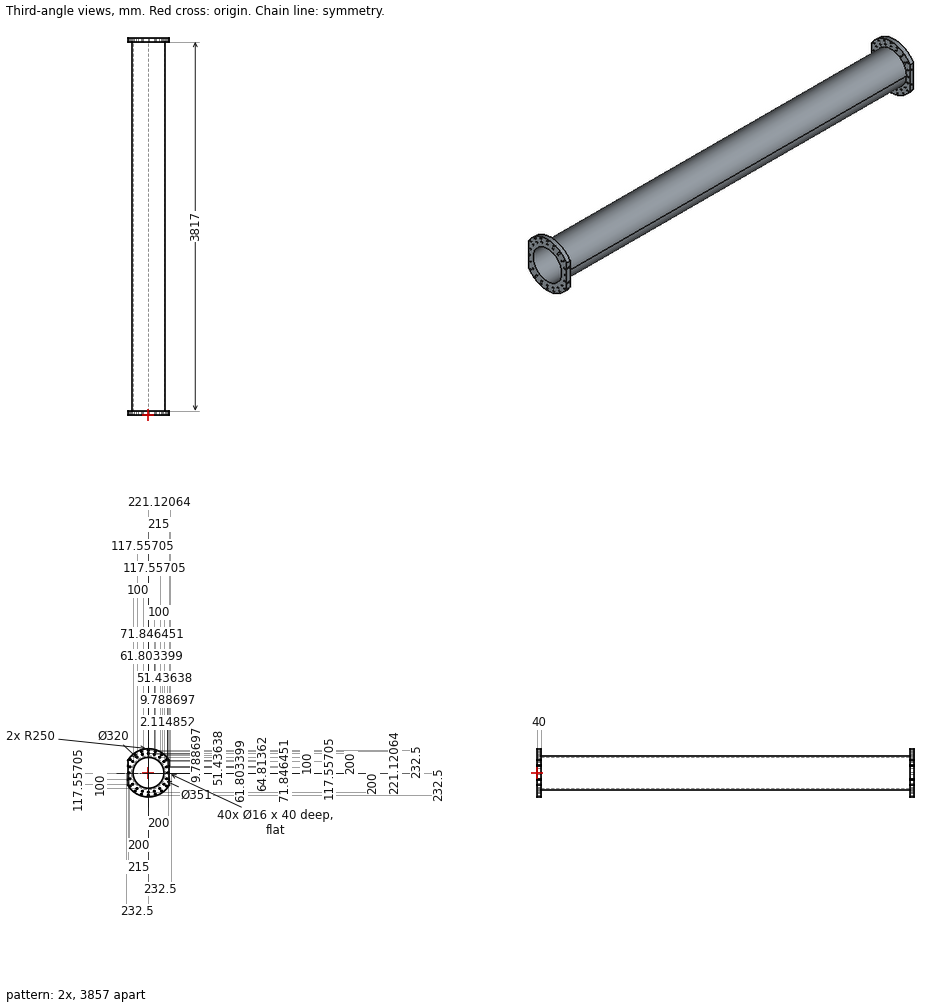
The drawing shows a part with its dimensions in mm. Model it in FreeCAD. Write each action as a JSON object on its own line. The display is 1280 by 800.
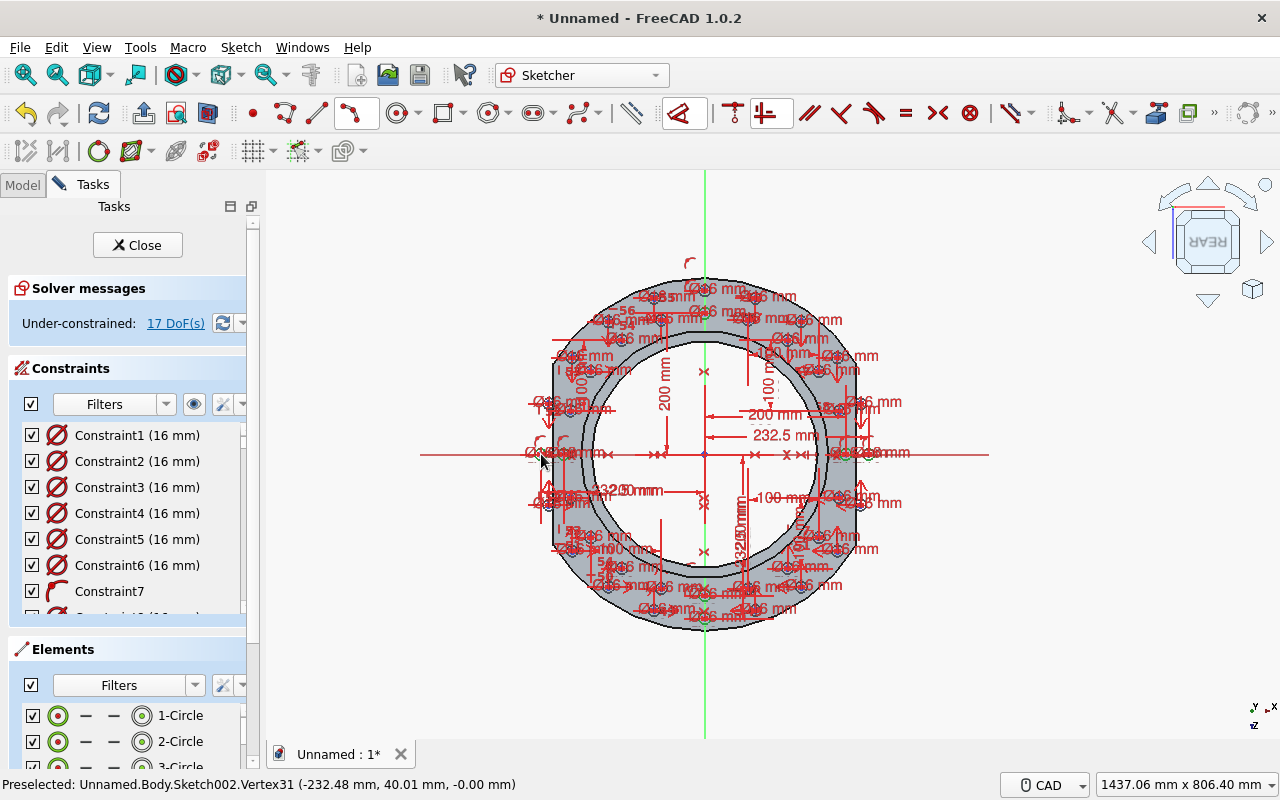
{"action": "left_click", "coordinate": [705, 291]}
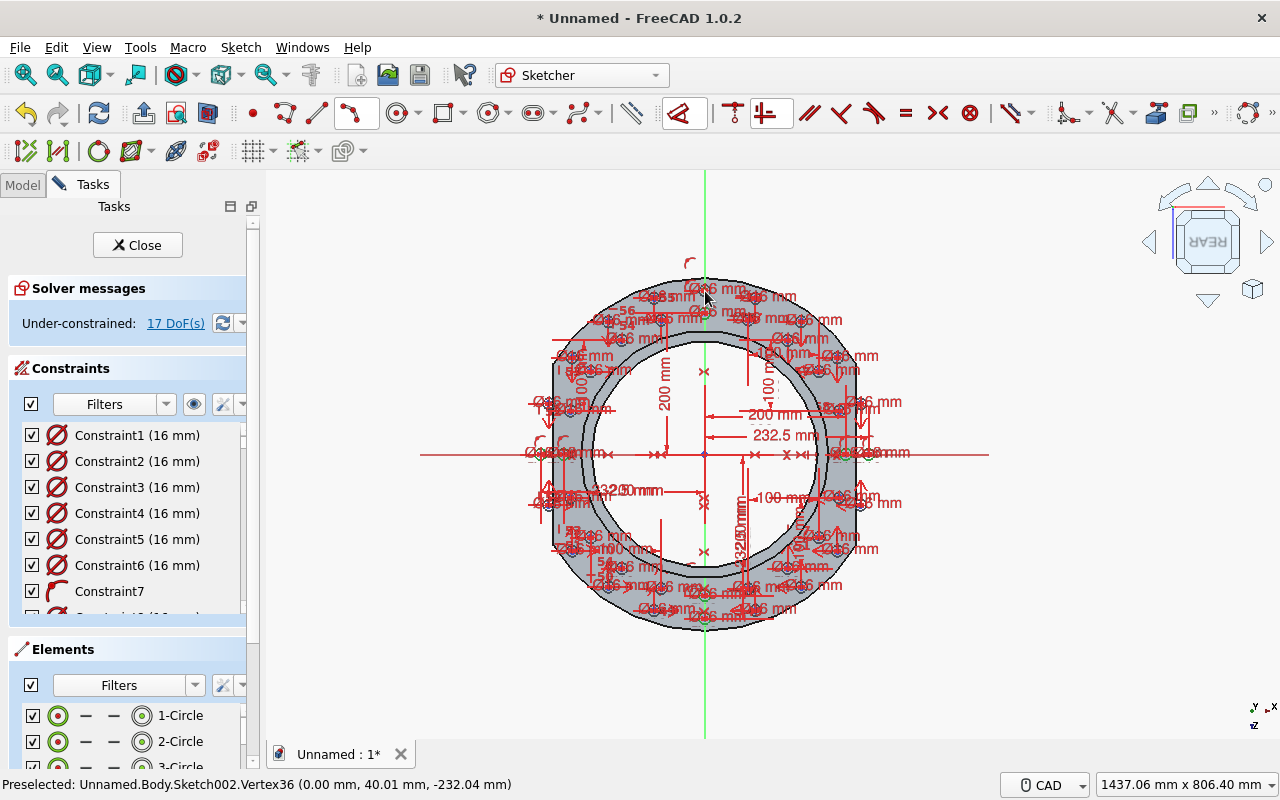
{"action": "key", "text": "i"}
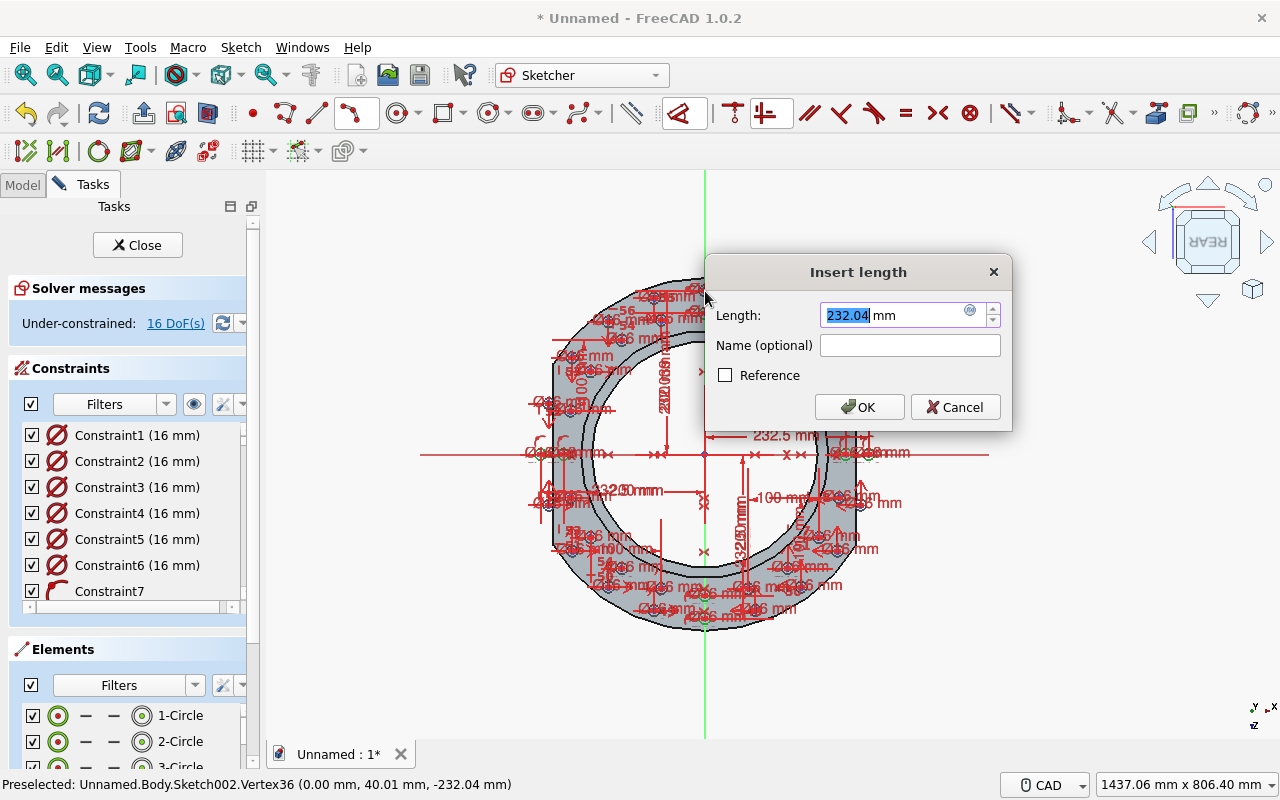
{"action": "type", "text": "232.5"}
{"action": "key", "text": "Return"}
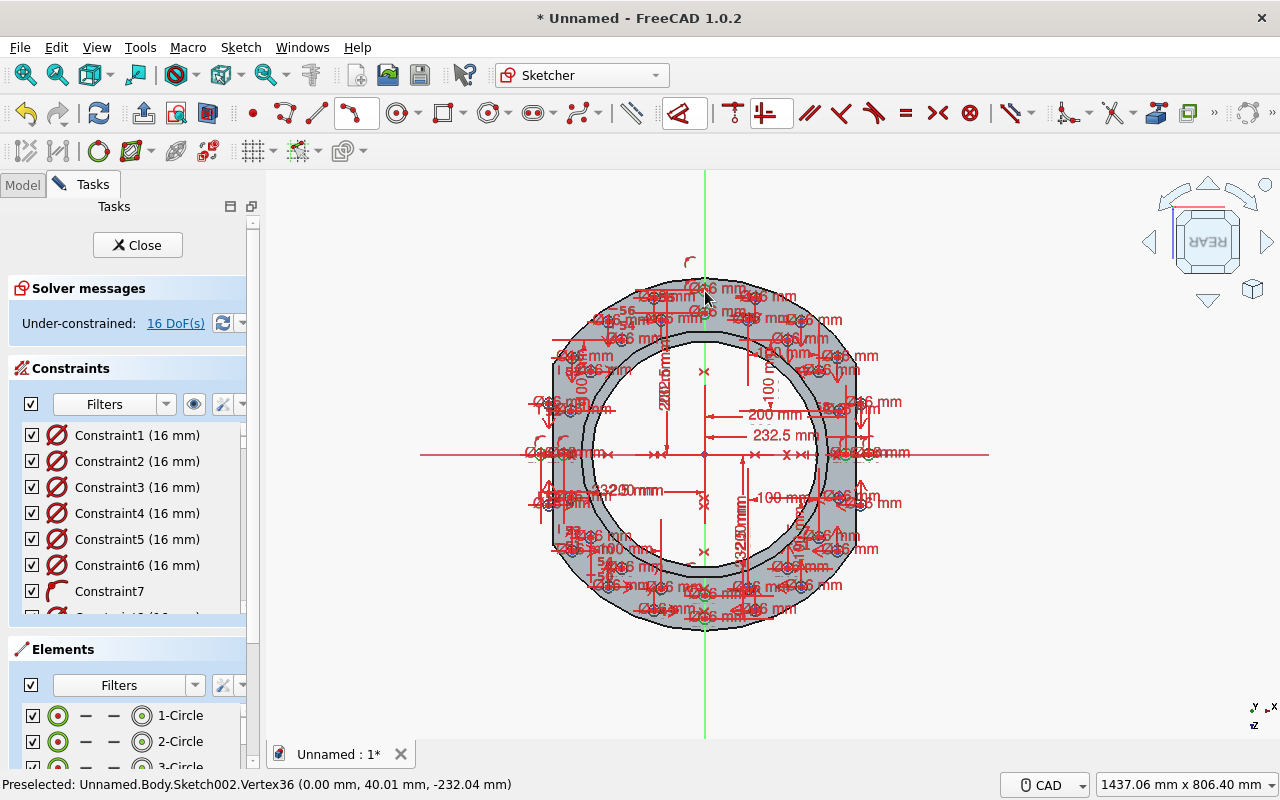
{"action": "left_click", "coordinate": [839, 498]}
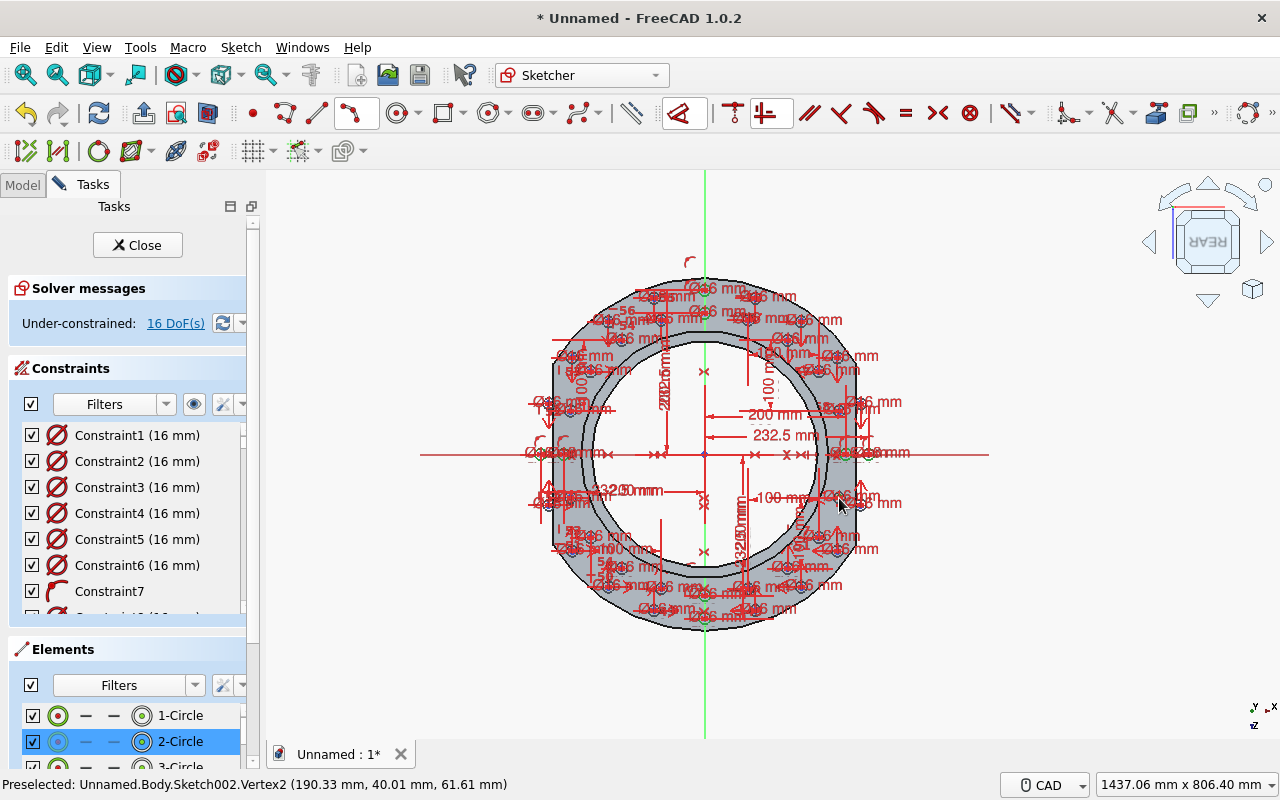
{"action": "key", "text": "i"}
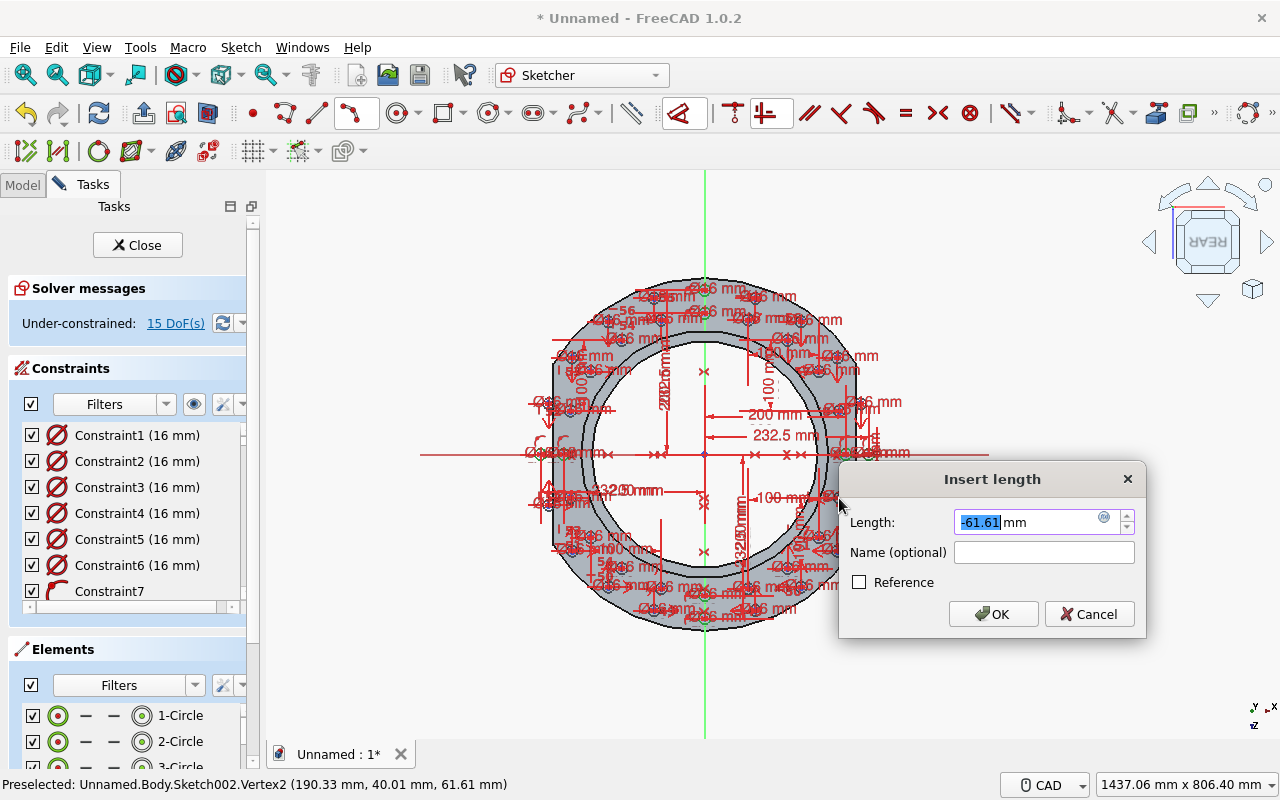
{"action": "type", "text": "-61.803399"}
{"action": "key", "text": "Return"}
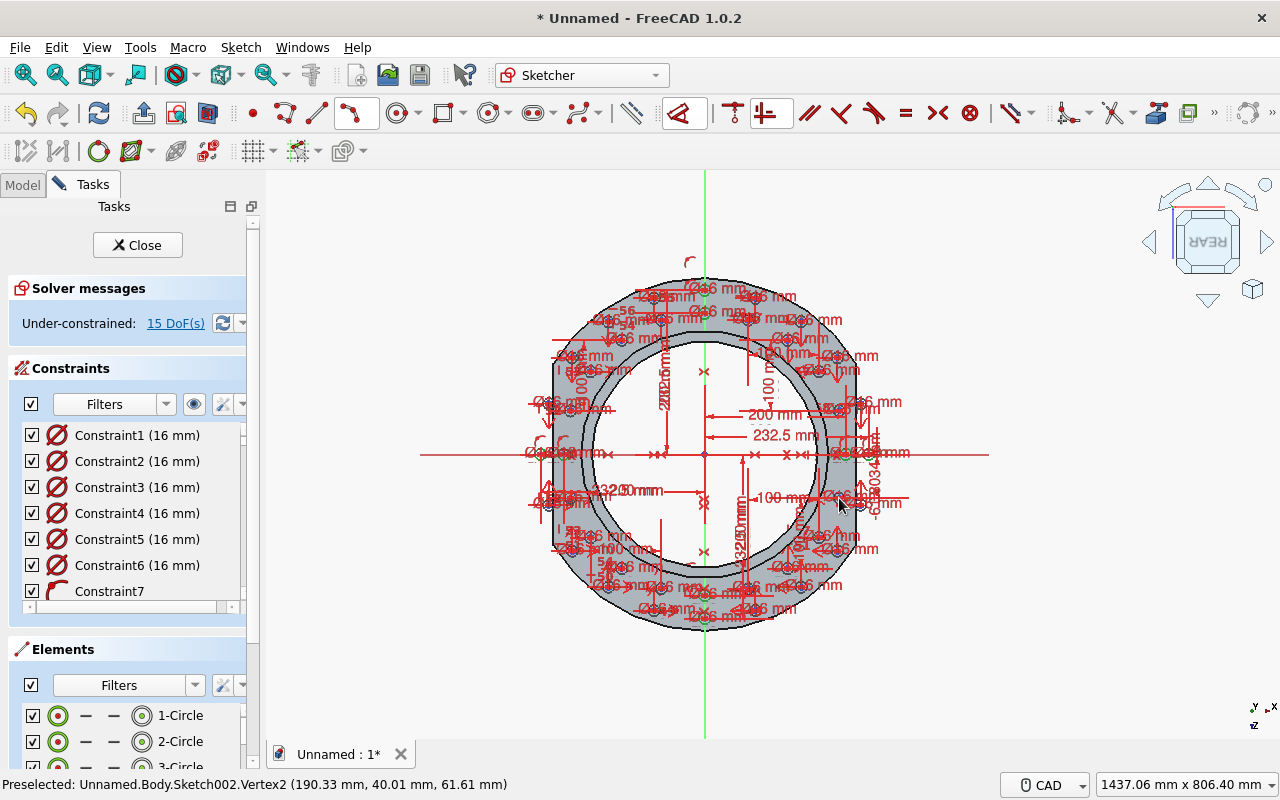
{"action": "left_click", "coordinate": [819, 538]}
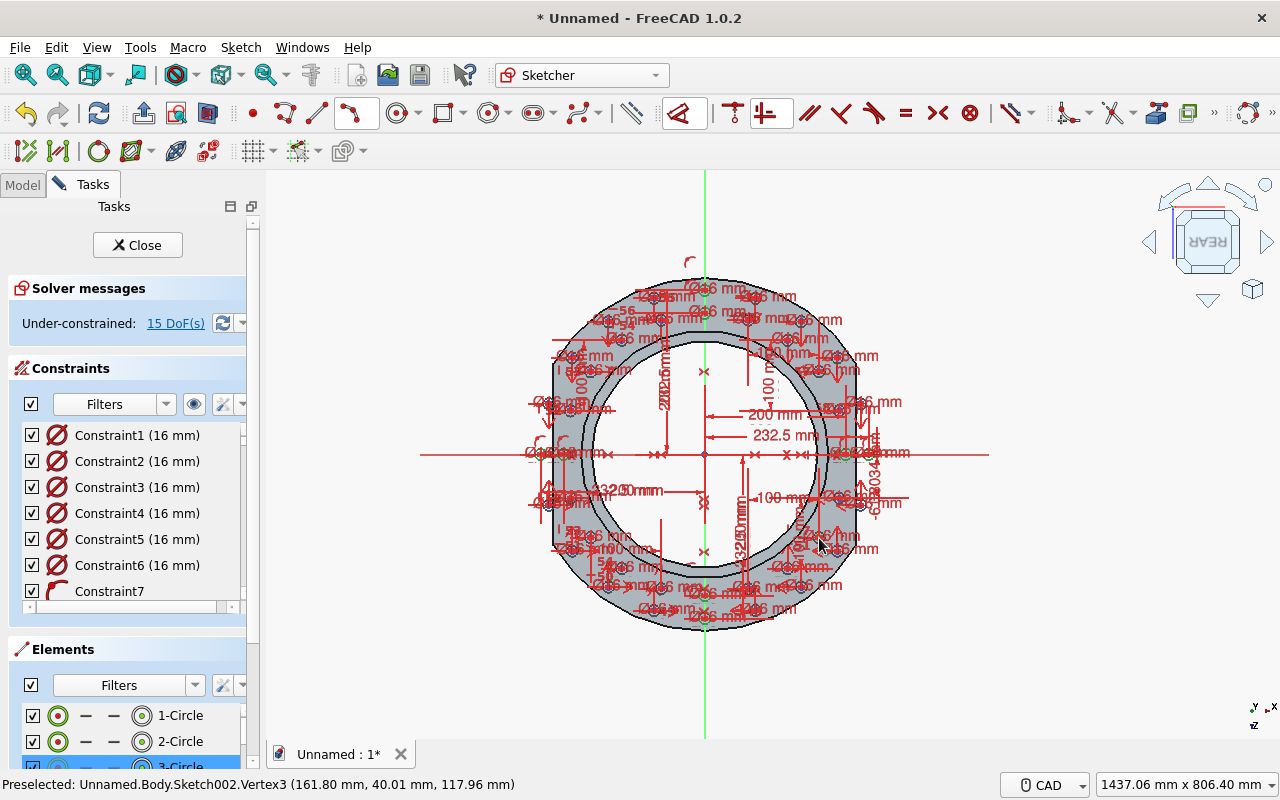
{"action": "key", "text": "i"}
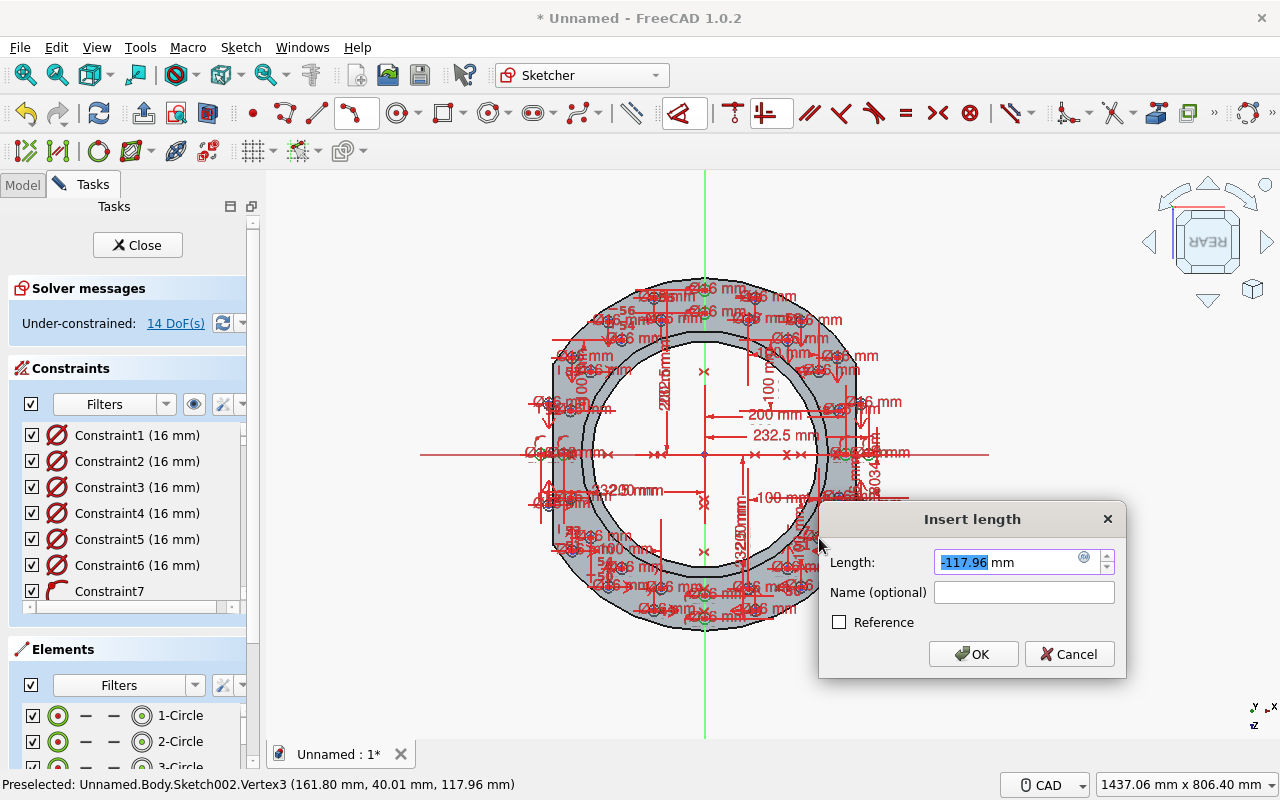
{"action": "type", "text": "-117.55705"}
{"action": "key", "text": "Return"}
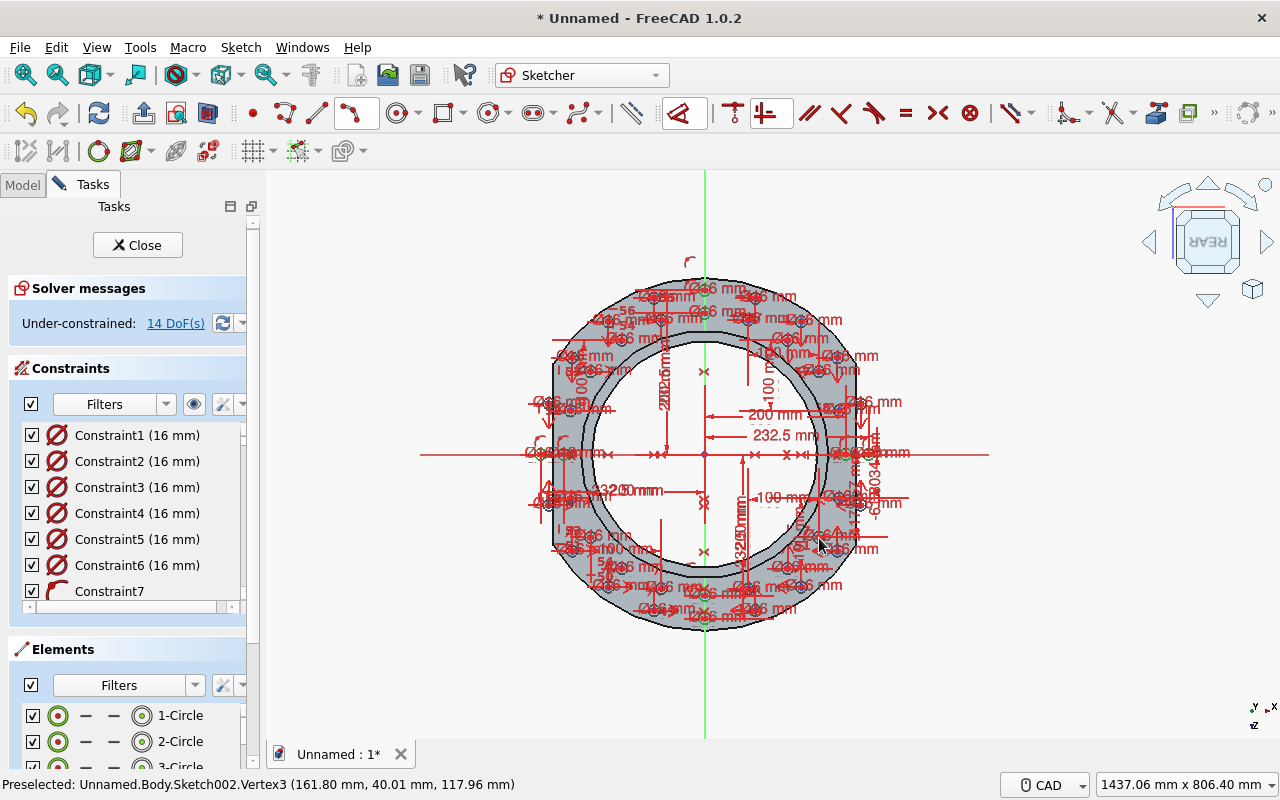
{"action": "left_click", "coordinate": [788, 569]}